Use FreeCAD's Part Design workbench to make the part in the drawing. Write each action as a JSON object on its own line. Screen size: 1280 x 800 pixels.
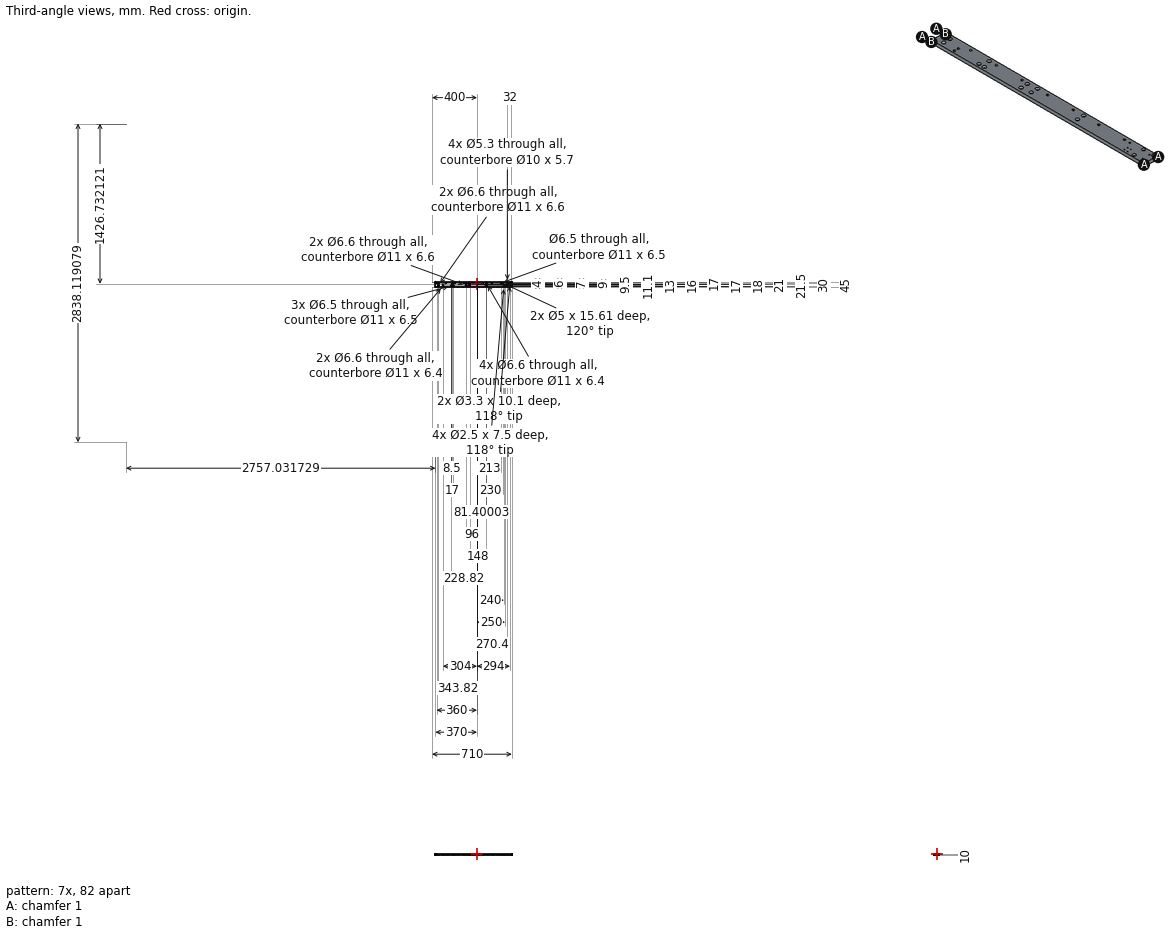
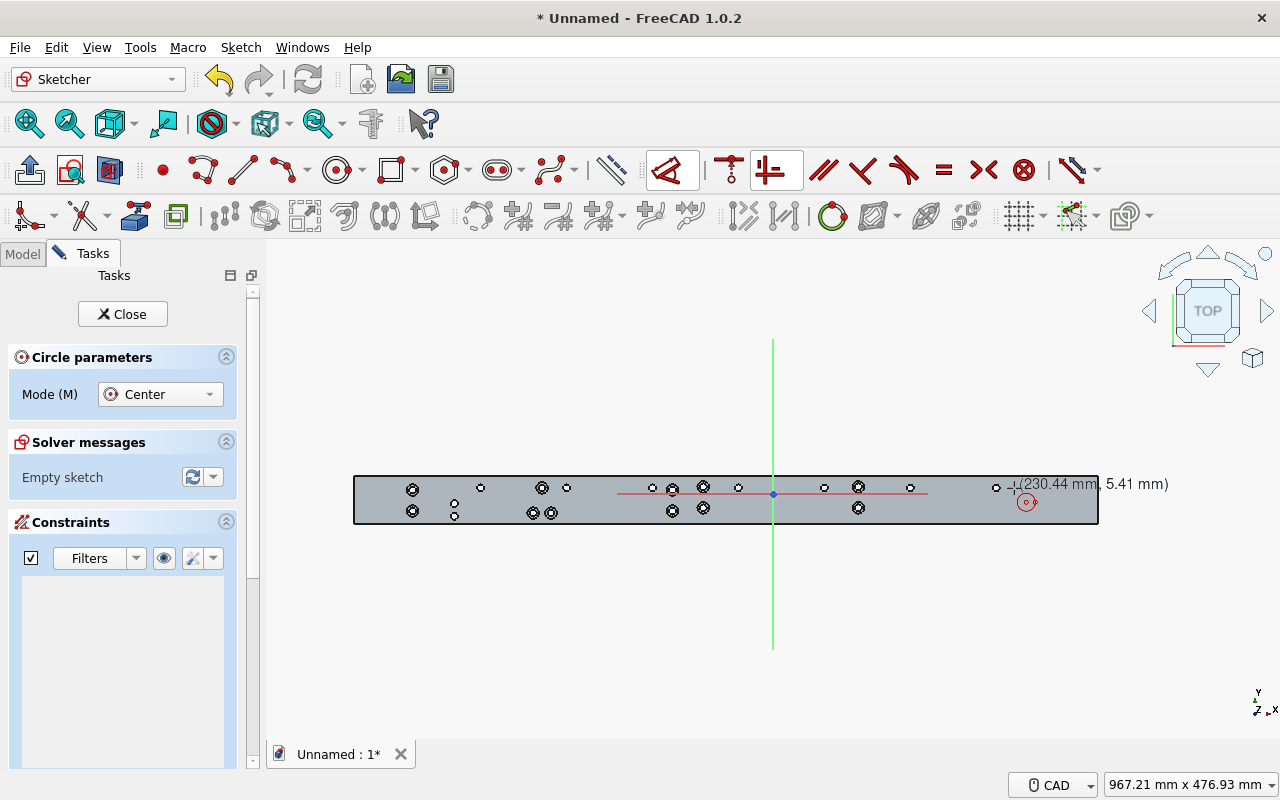
{"action": "scroll", "coordinate": [1014, 488], "scroll_direction": "up", "scroll_amount": 5}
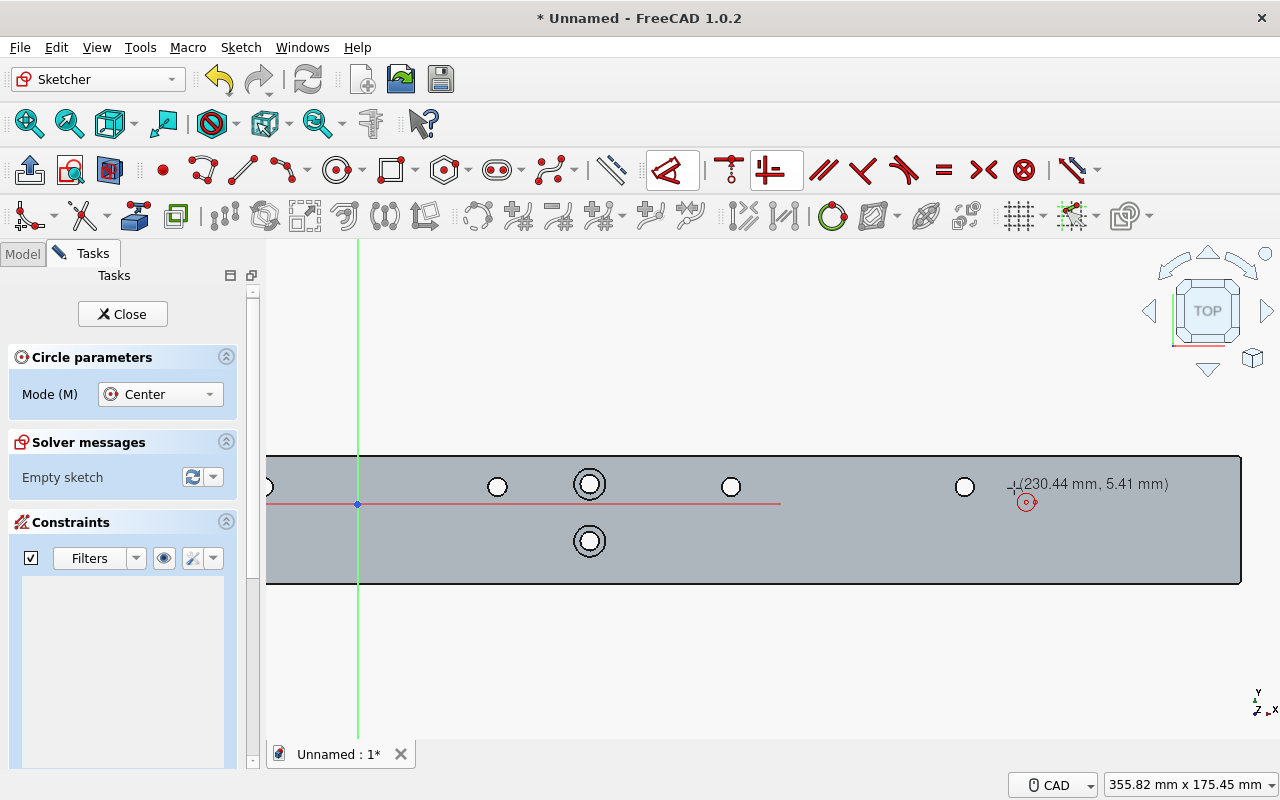
{"action": "left_click", "coordinate": [1013, 487]}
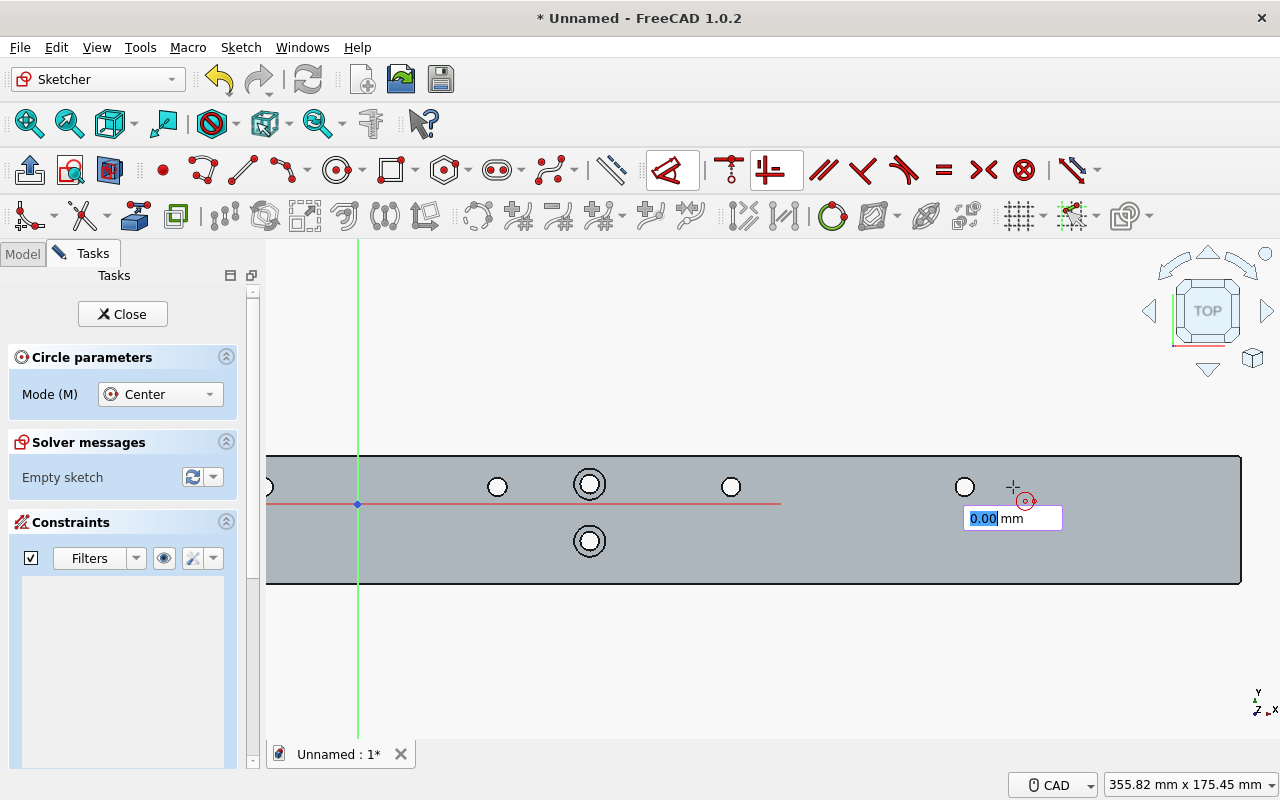
{"action": "scroll", "coordinate": [1018, 482], "scroll_direction": "up", "scroll_amount": 5}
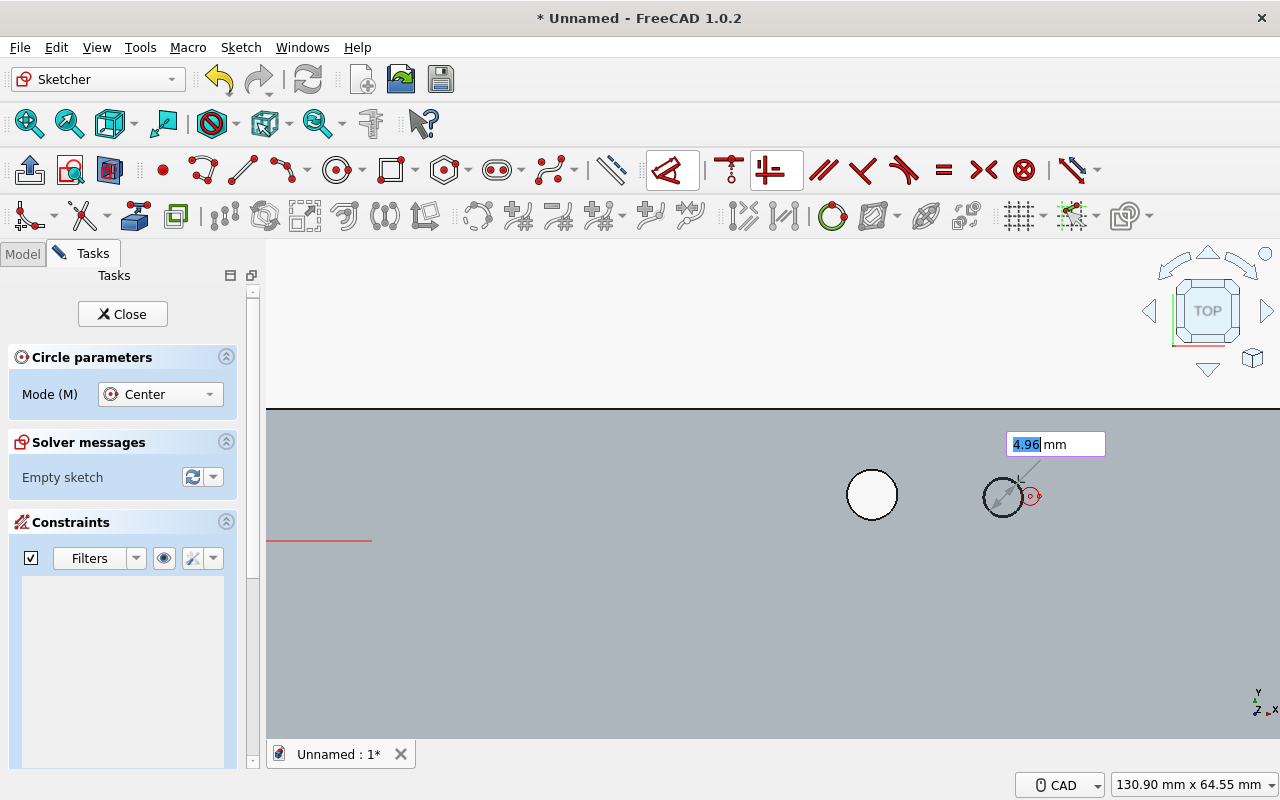
{"action": "left_click", "coordinate": [1018, 481]}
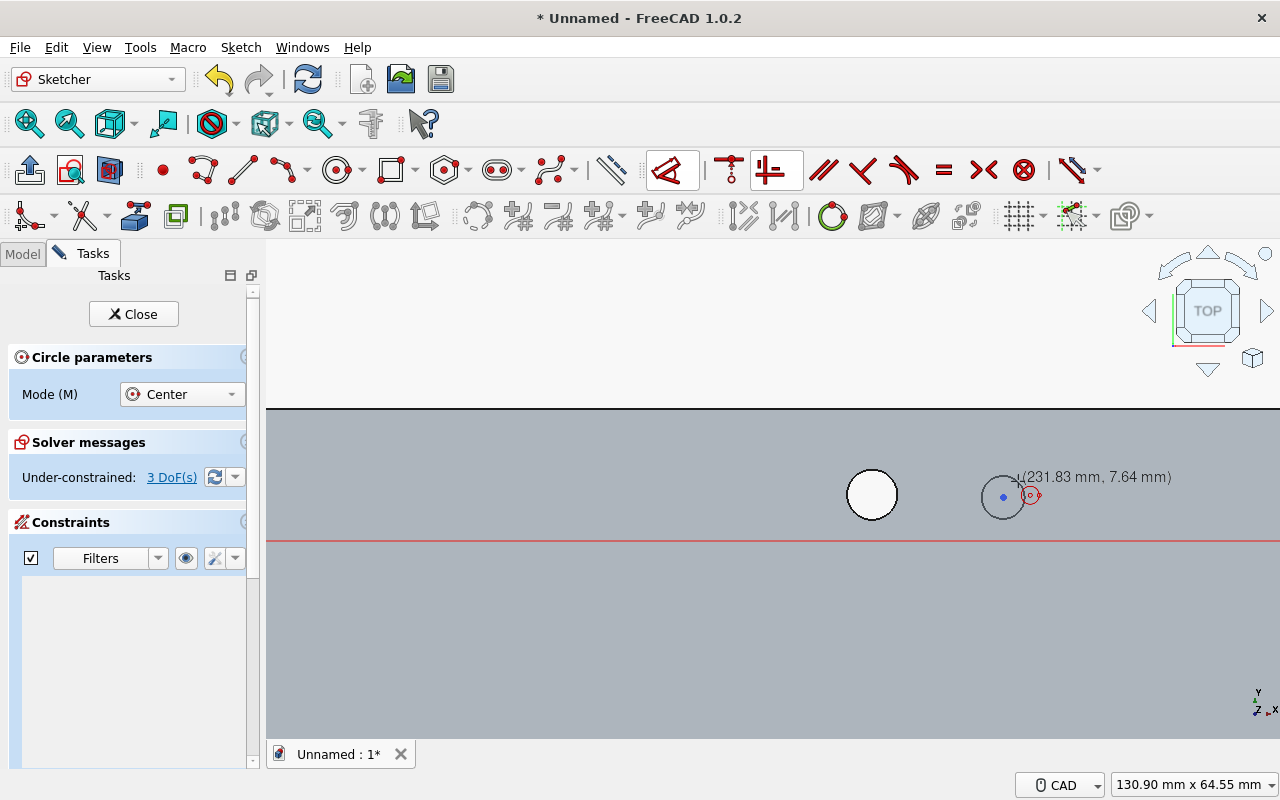
{"action": "scroll", "coordinate": [1015, 486], "scroll_direction": "down", "scroll_amount": 10}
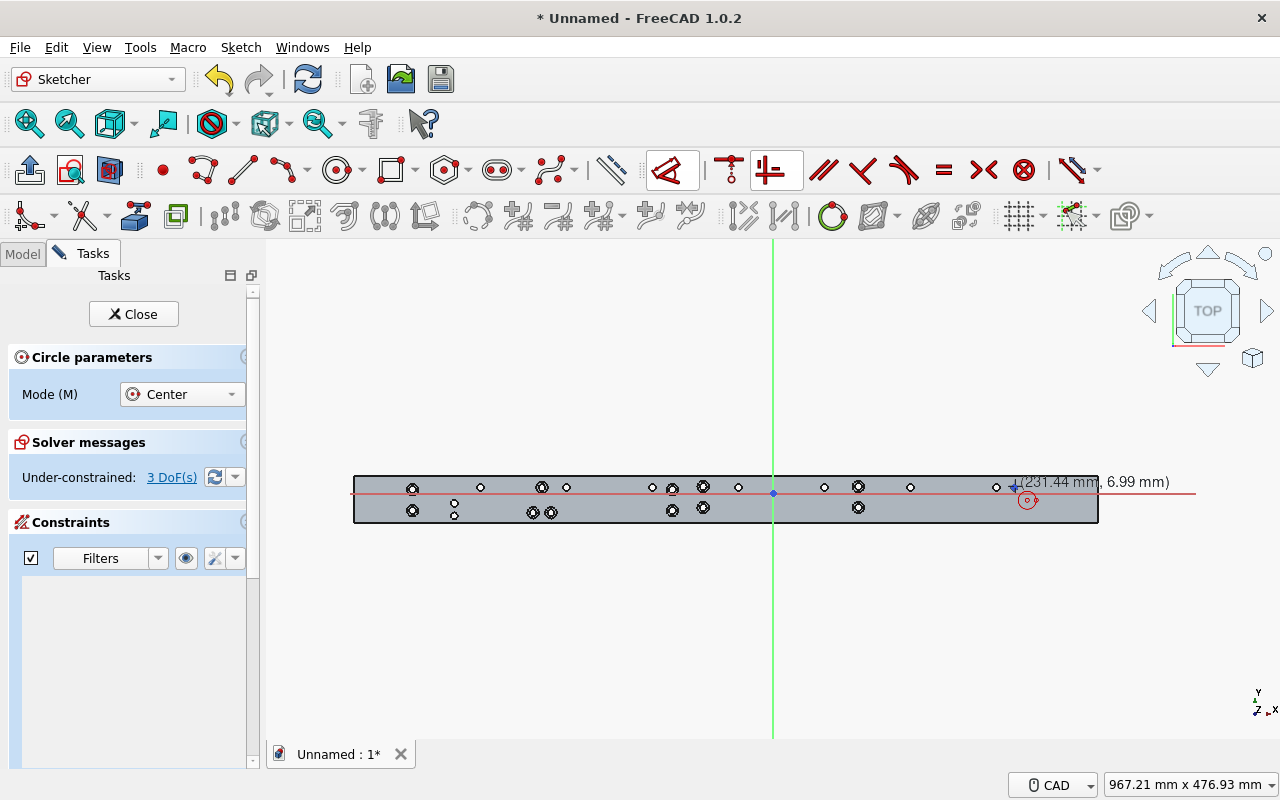
{"action": "scroll", "coordinate": [396, 488], "scroll_direction": "up", "scroll_amount": 11}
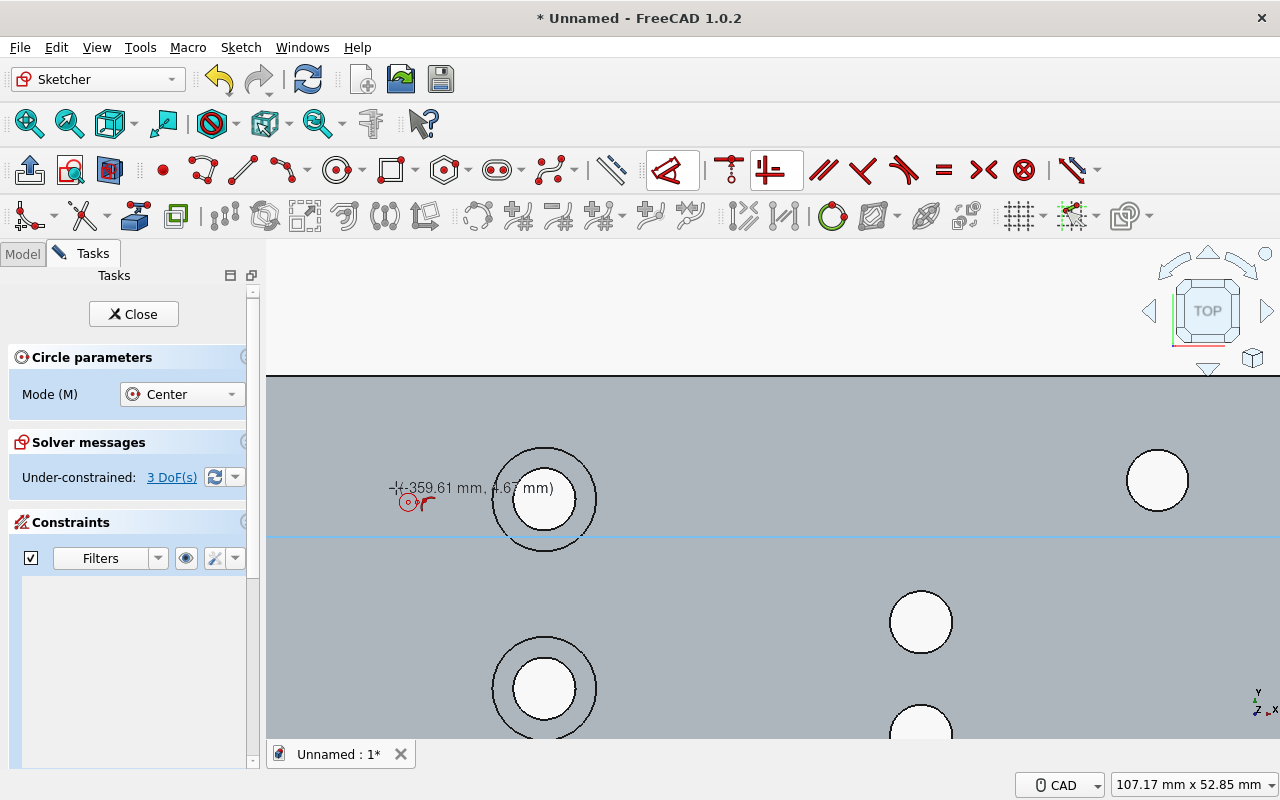
{"action": "scroll", "coordinate": [396, 488], "scroll_direction": "down", "scroll_amount": 11}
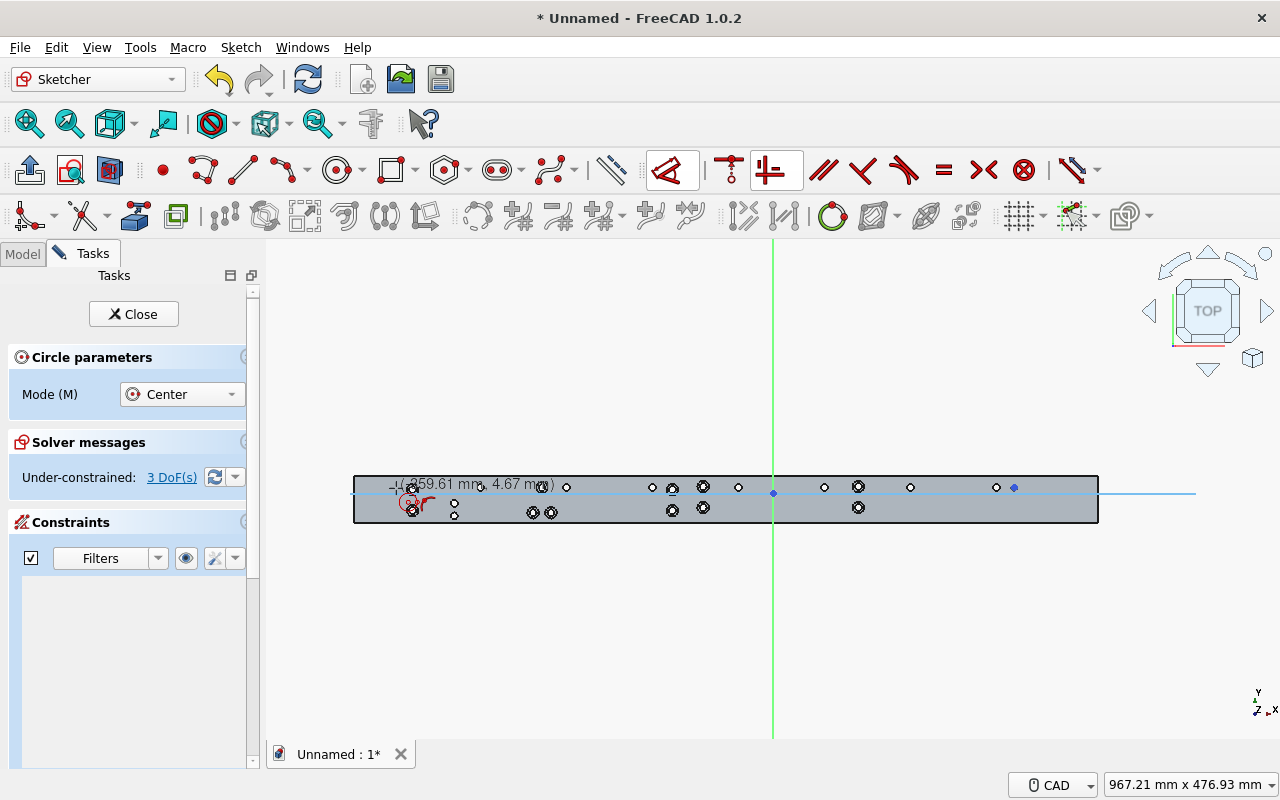
{"action": "scroll", "coordinate": [396, 488], "scroll_direction": "up", "scroll_amount": 5}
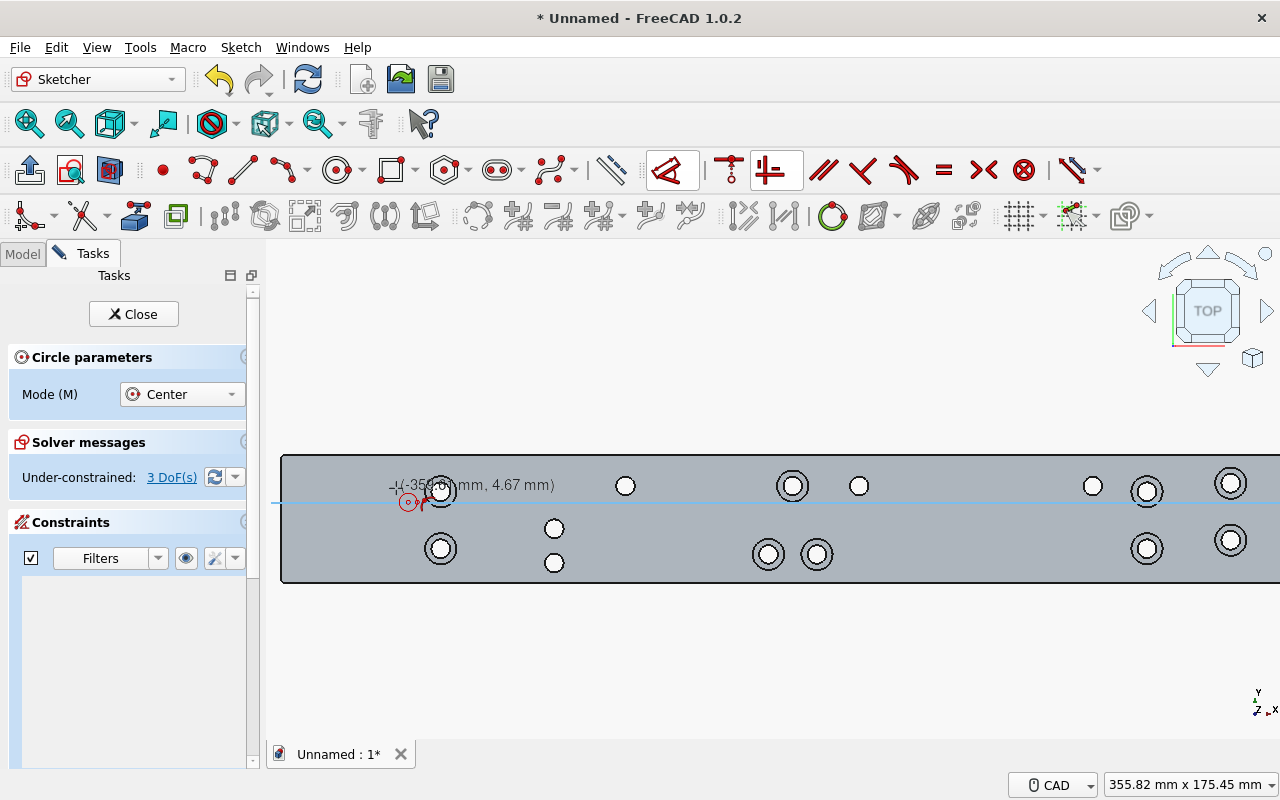
{"action": "left_click", "coordinate": [395, 486]}